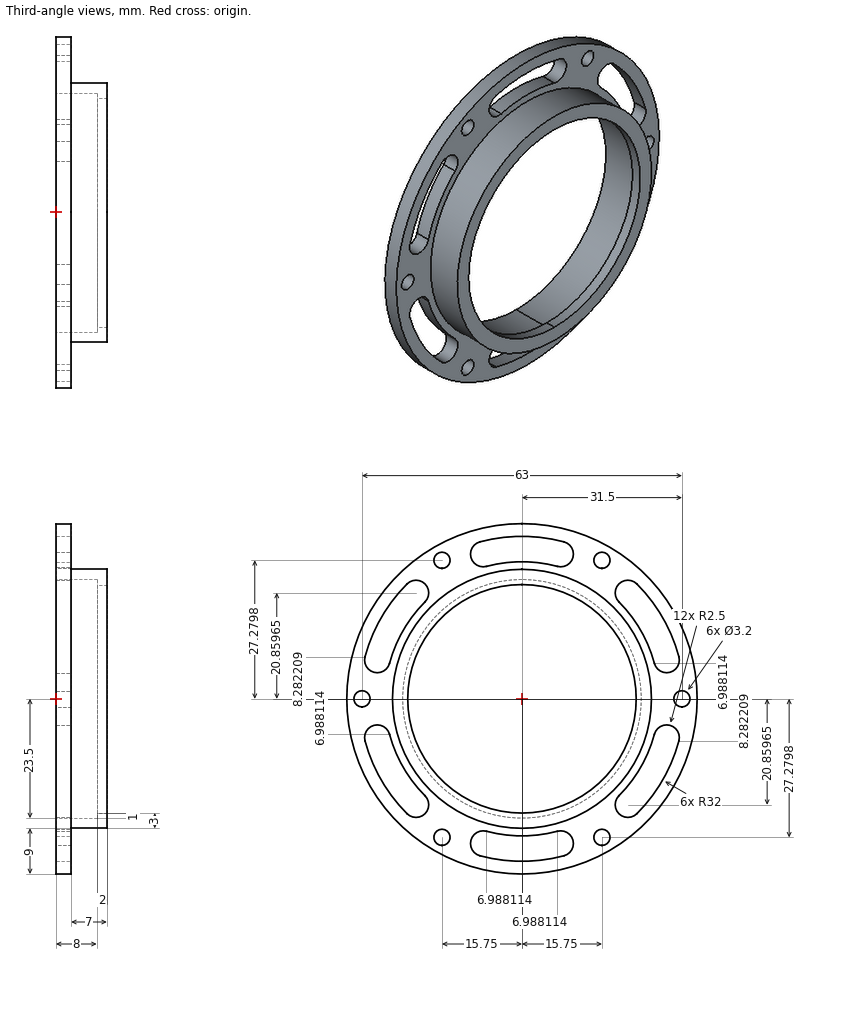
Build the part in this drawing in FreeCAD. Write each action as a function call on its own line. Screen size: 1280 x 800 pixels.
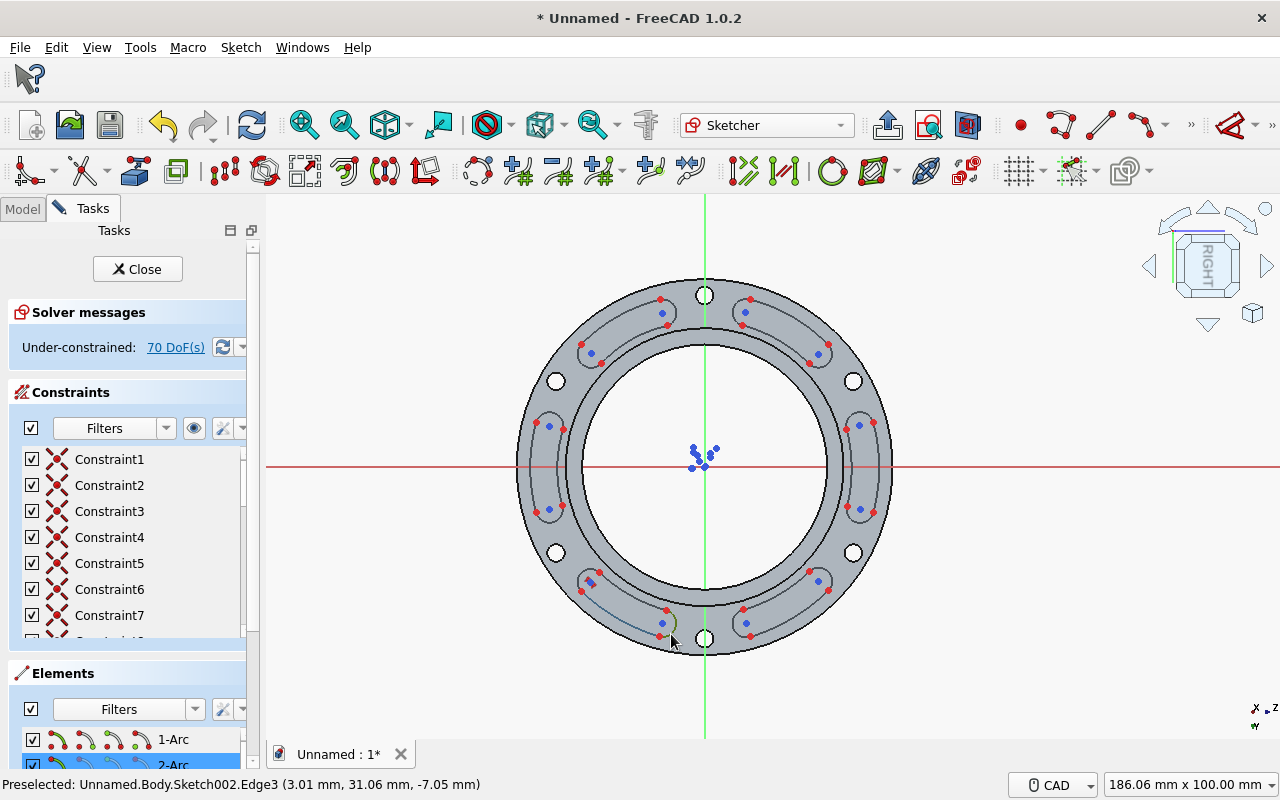
key(t)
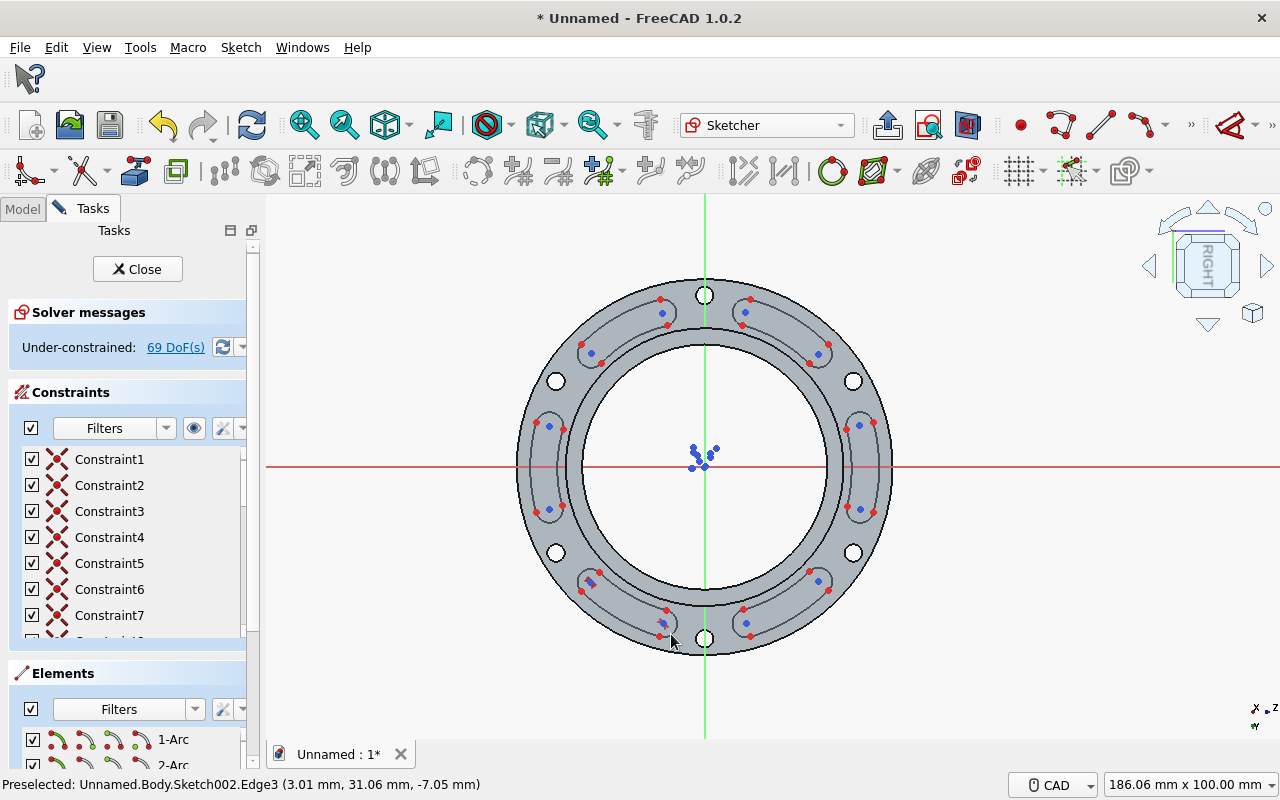
click(672, 634)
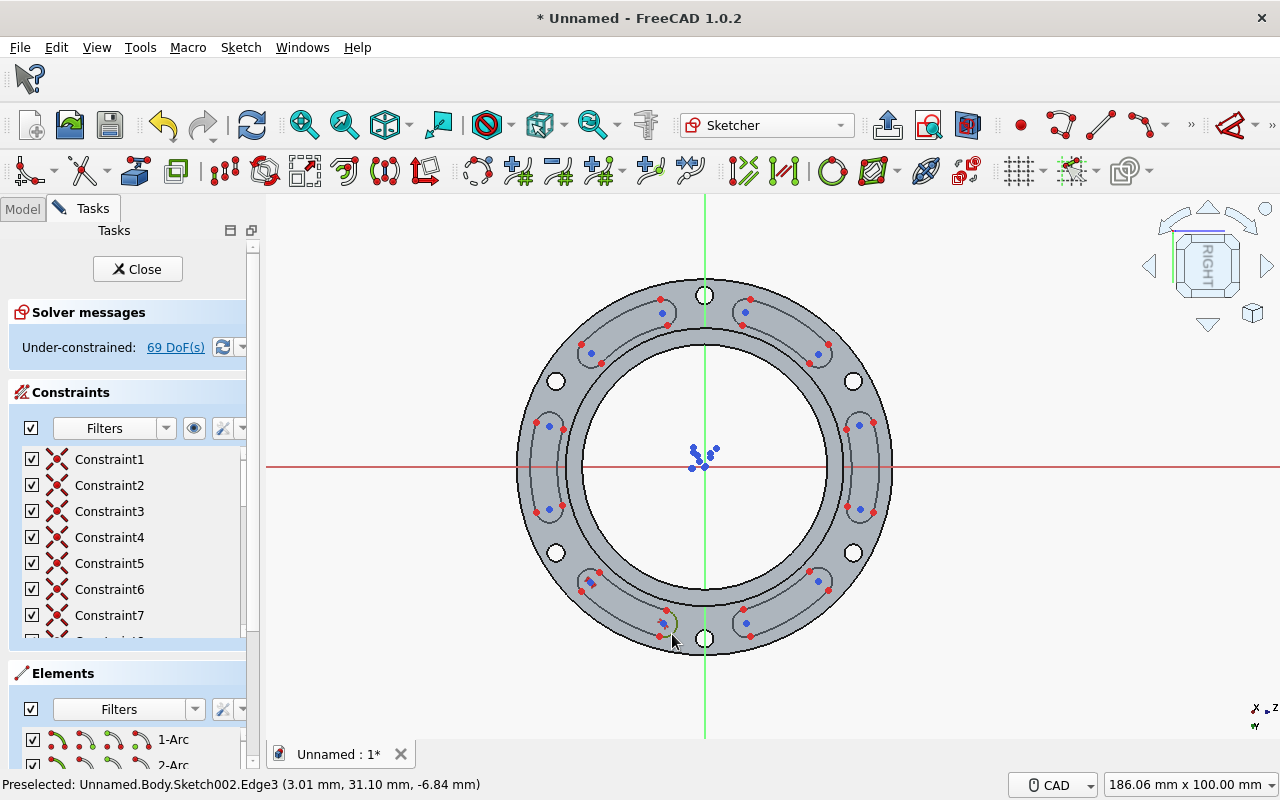
click(618, 587)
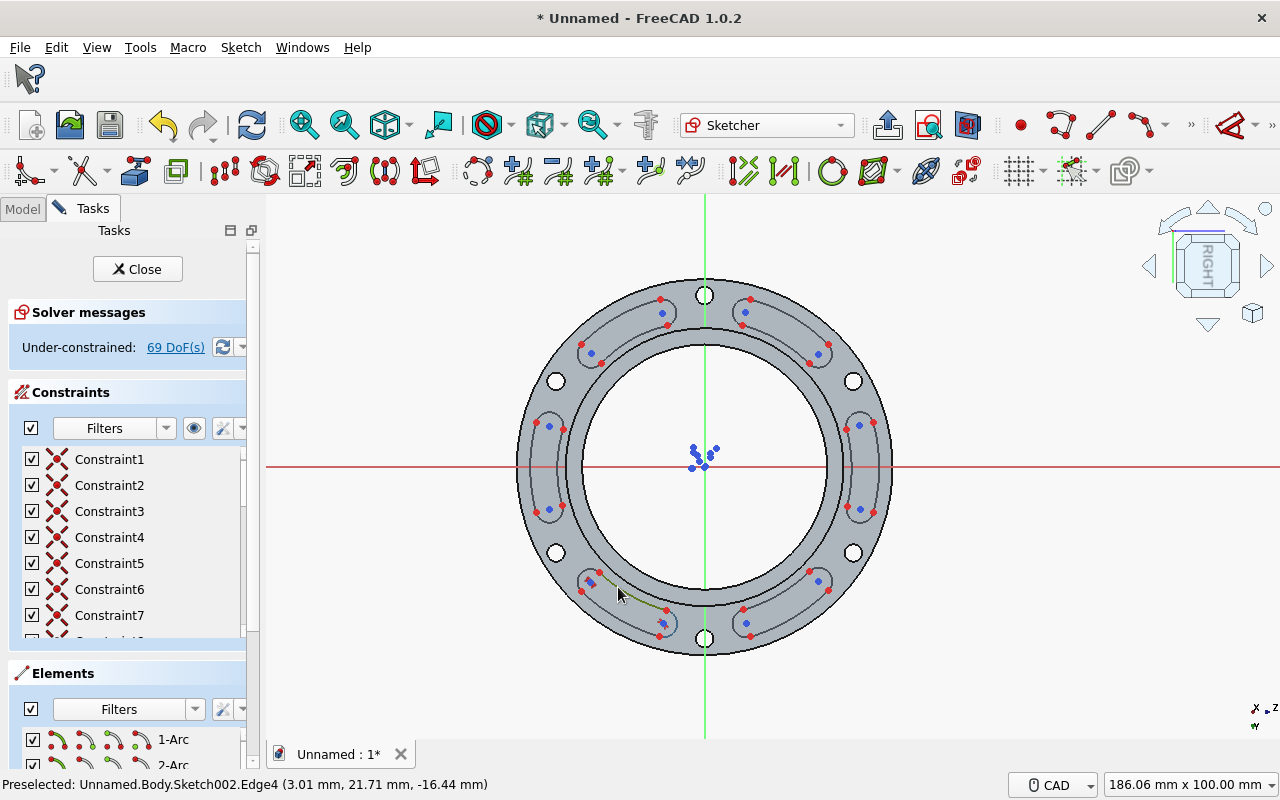
key(t)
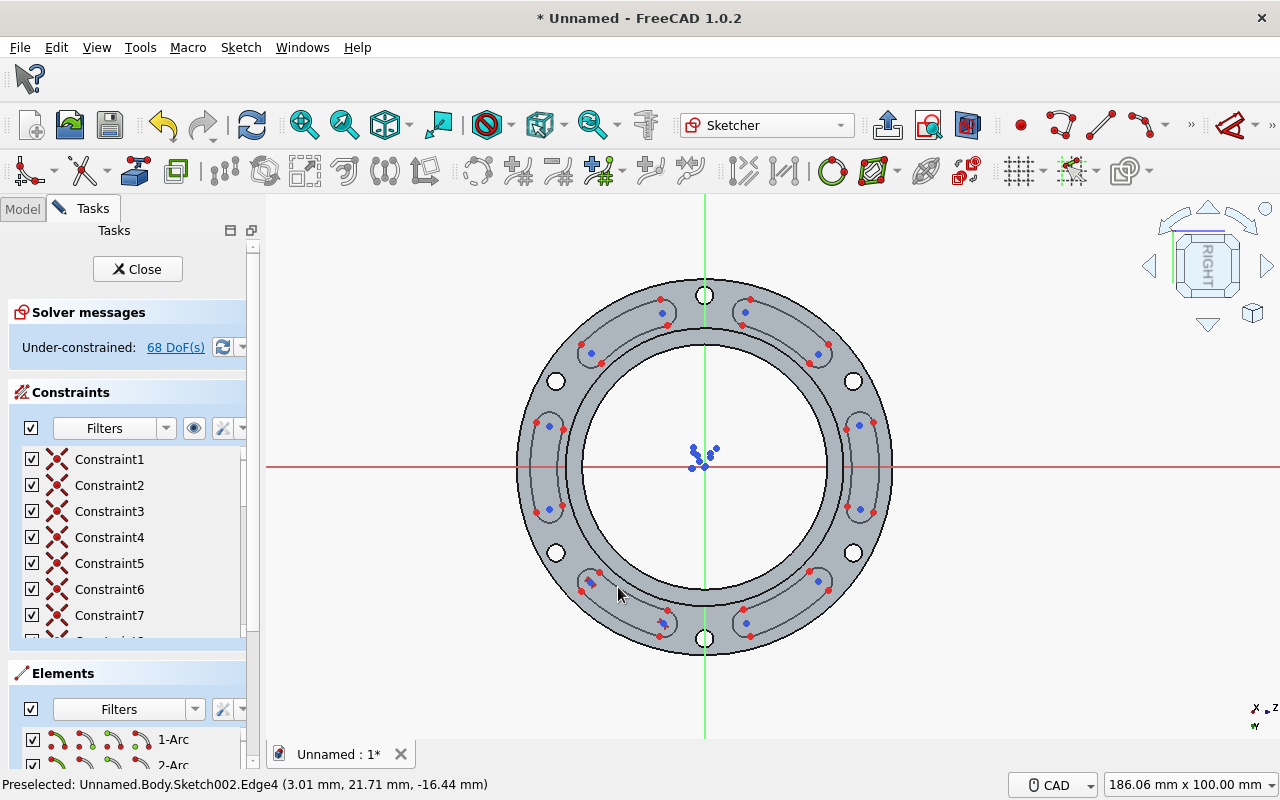
click(558, 452)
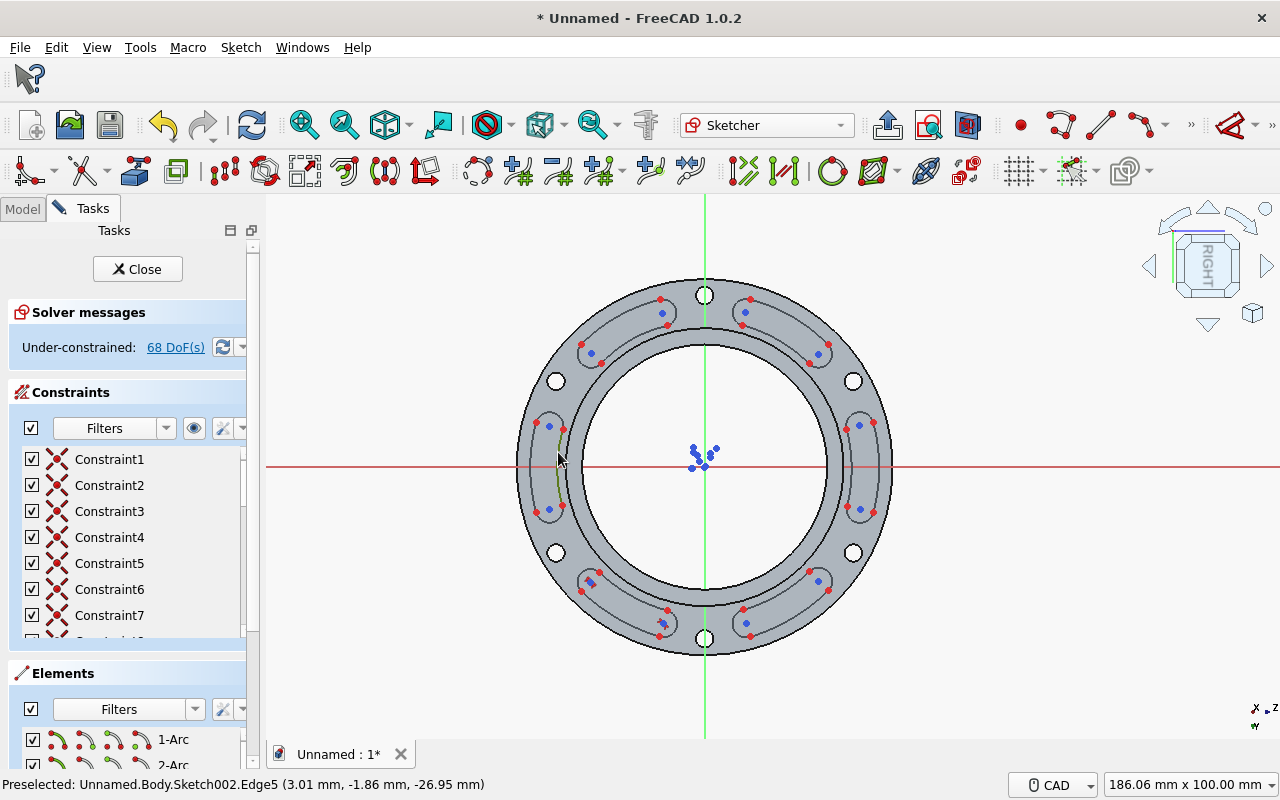
click(561, 418)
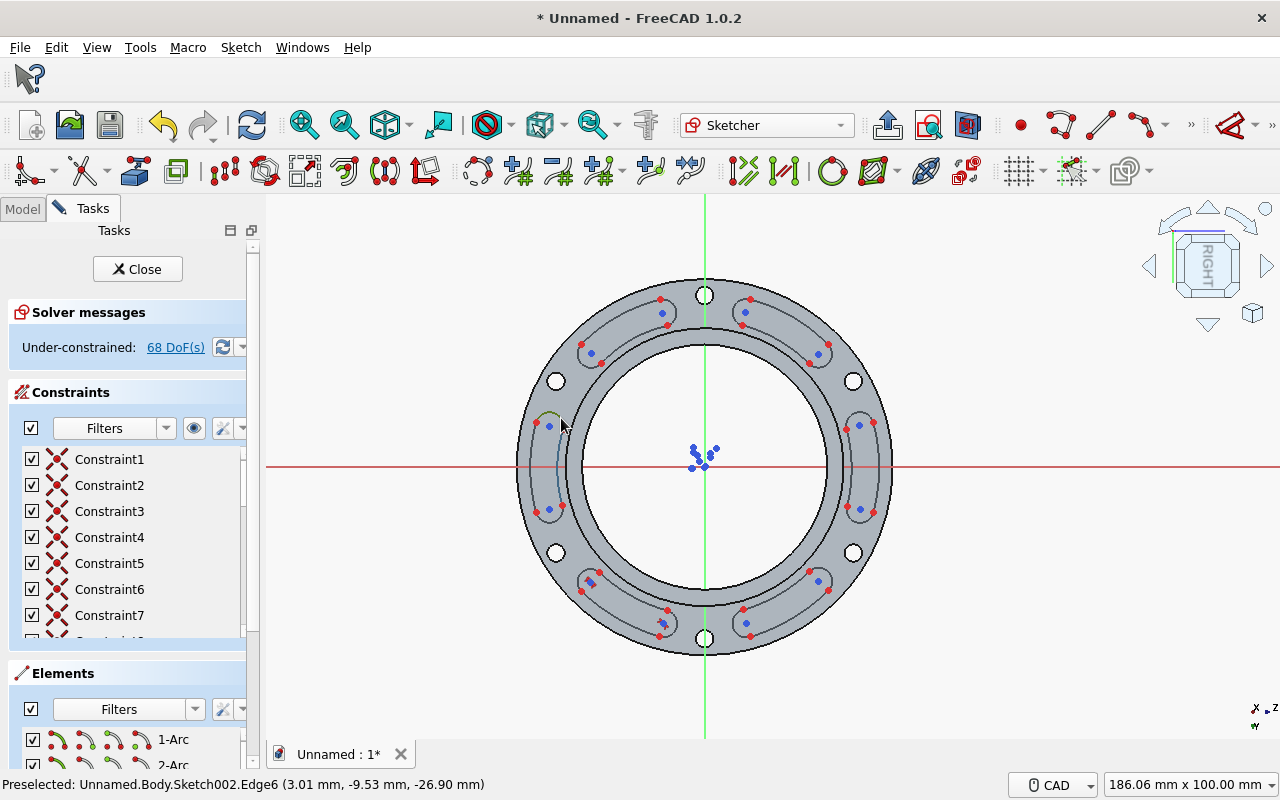
key(t)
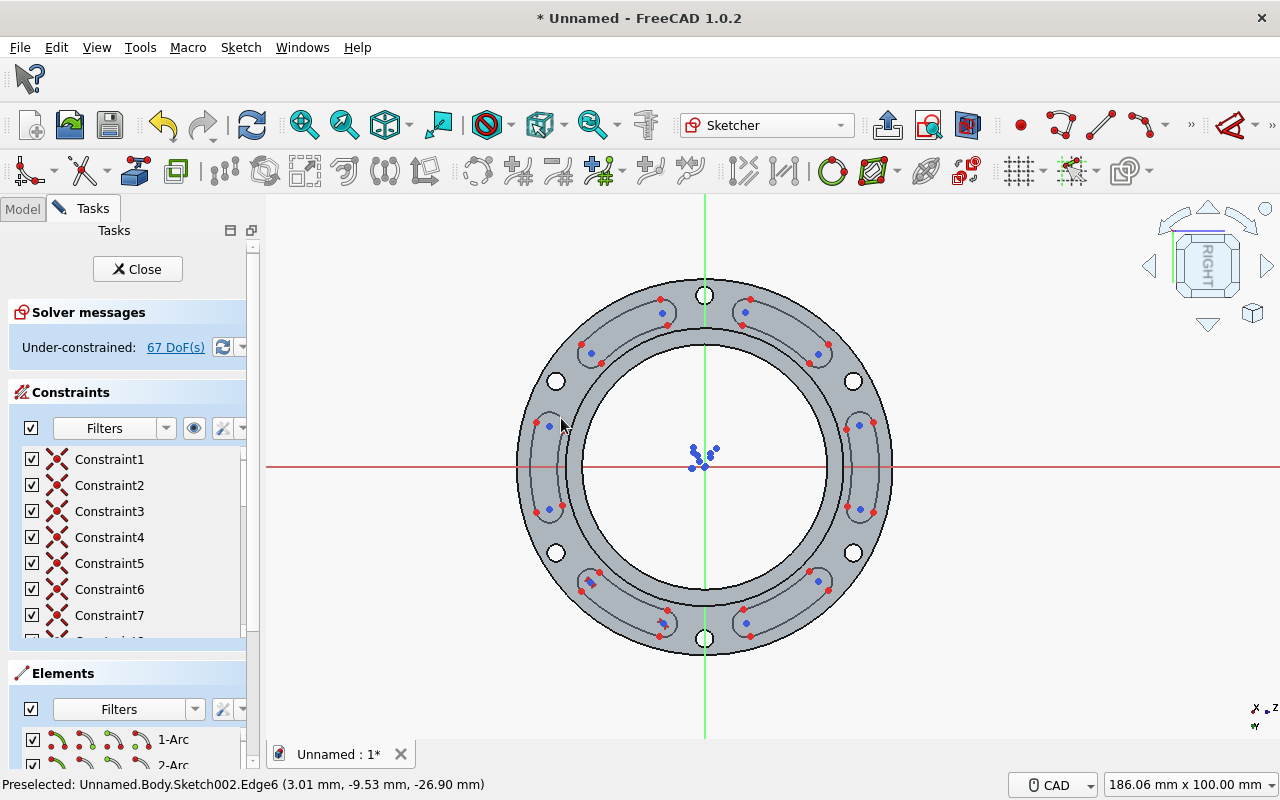
click(558, 453)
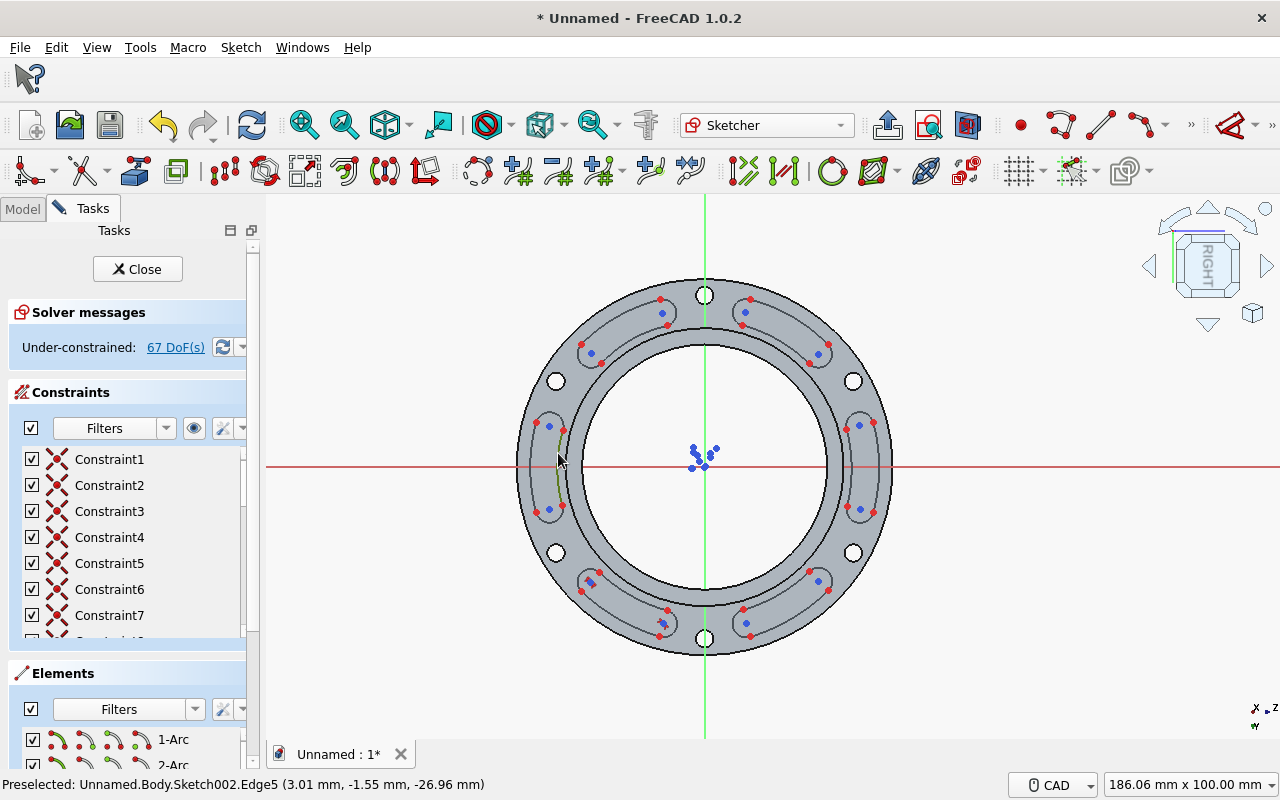
click(545, 522)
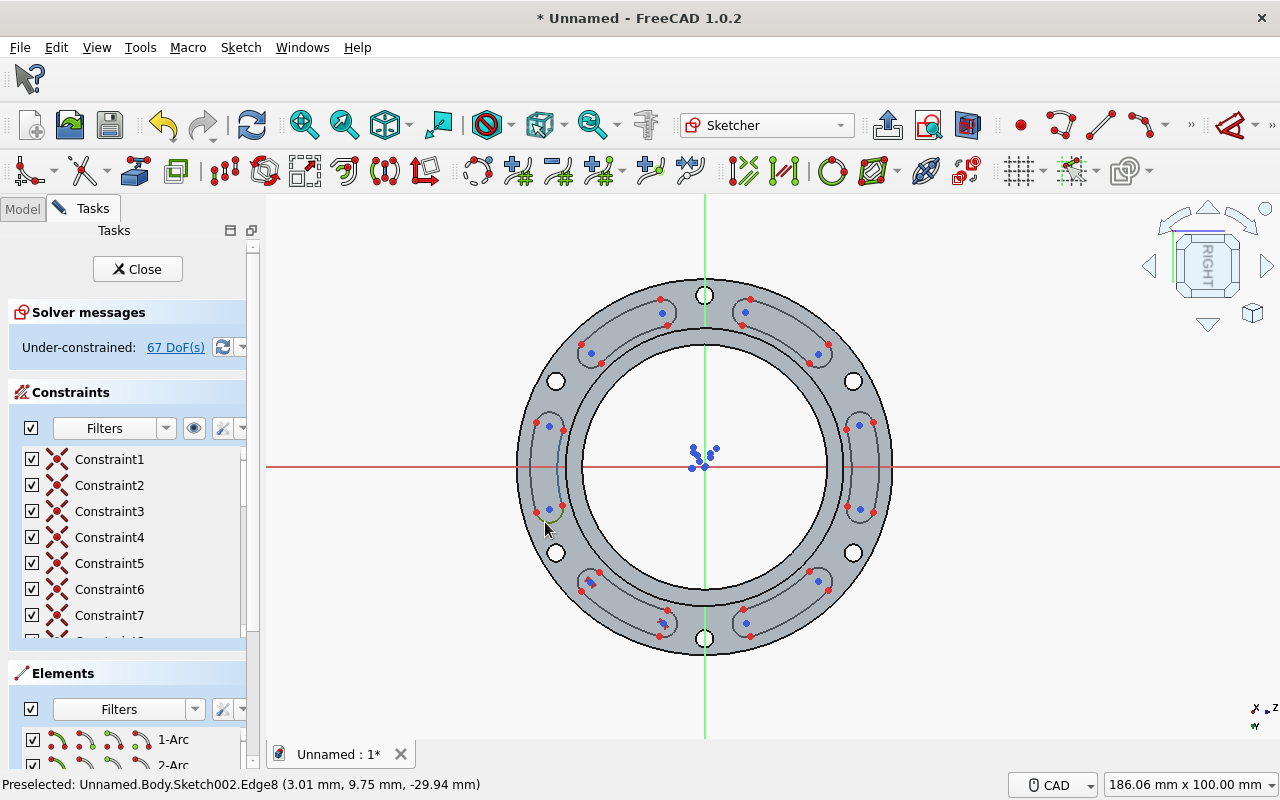
key(t)